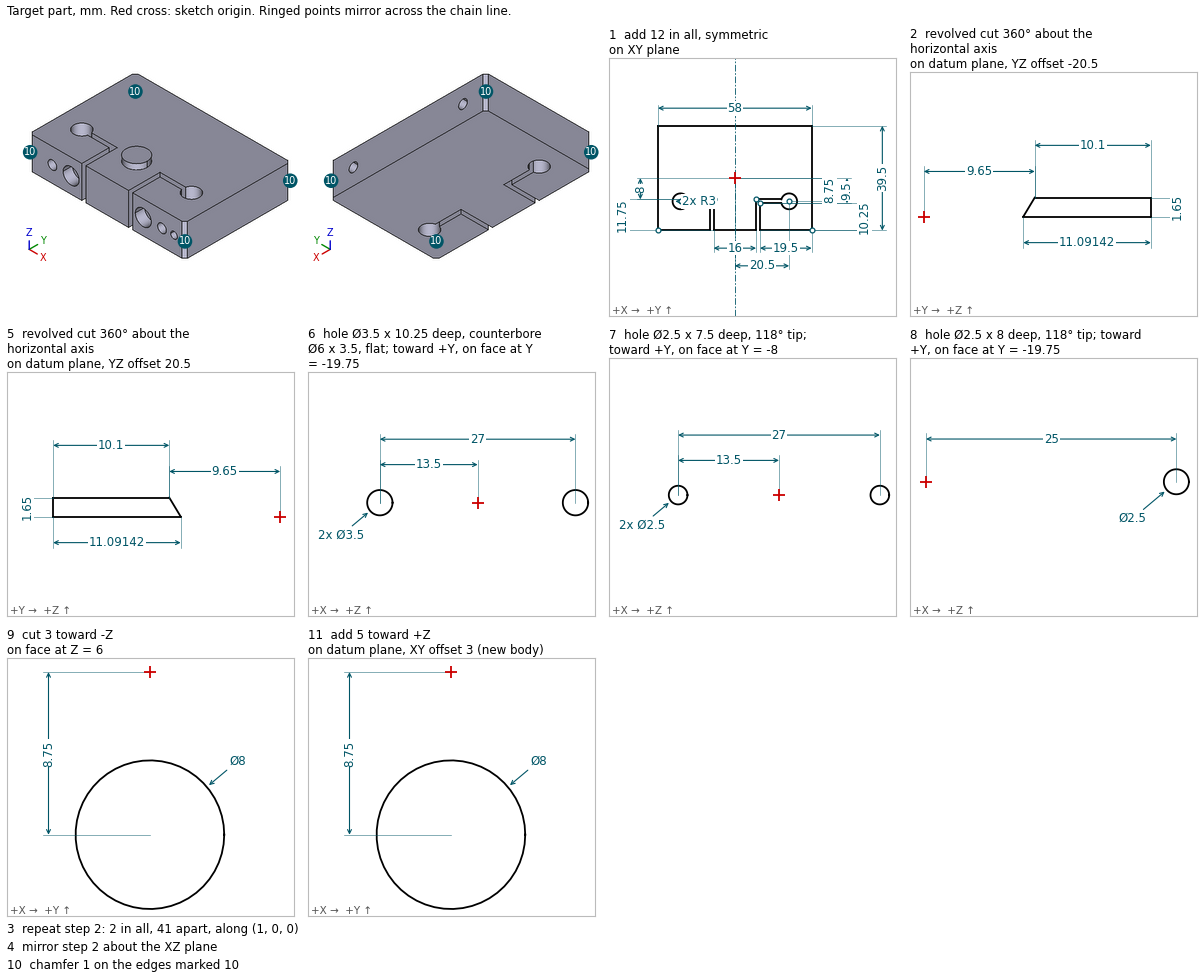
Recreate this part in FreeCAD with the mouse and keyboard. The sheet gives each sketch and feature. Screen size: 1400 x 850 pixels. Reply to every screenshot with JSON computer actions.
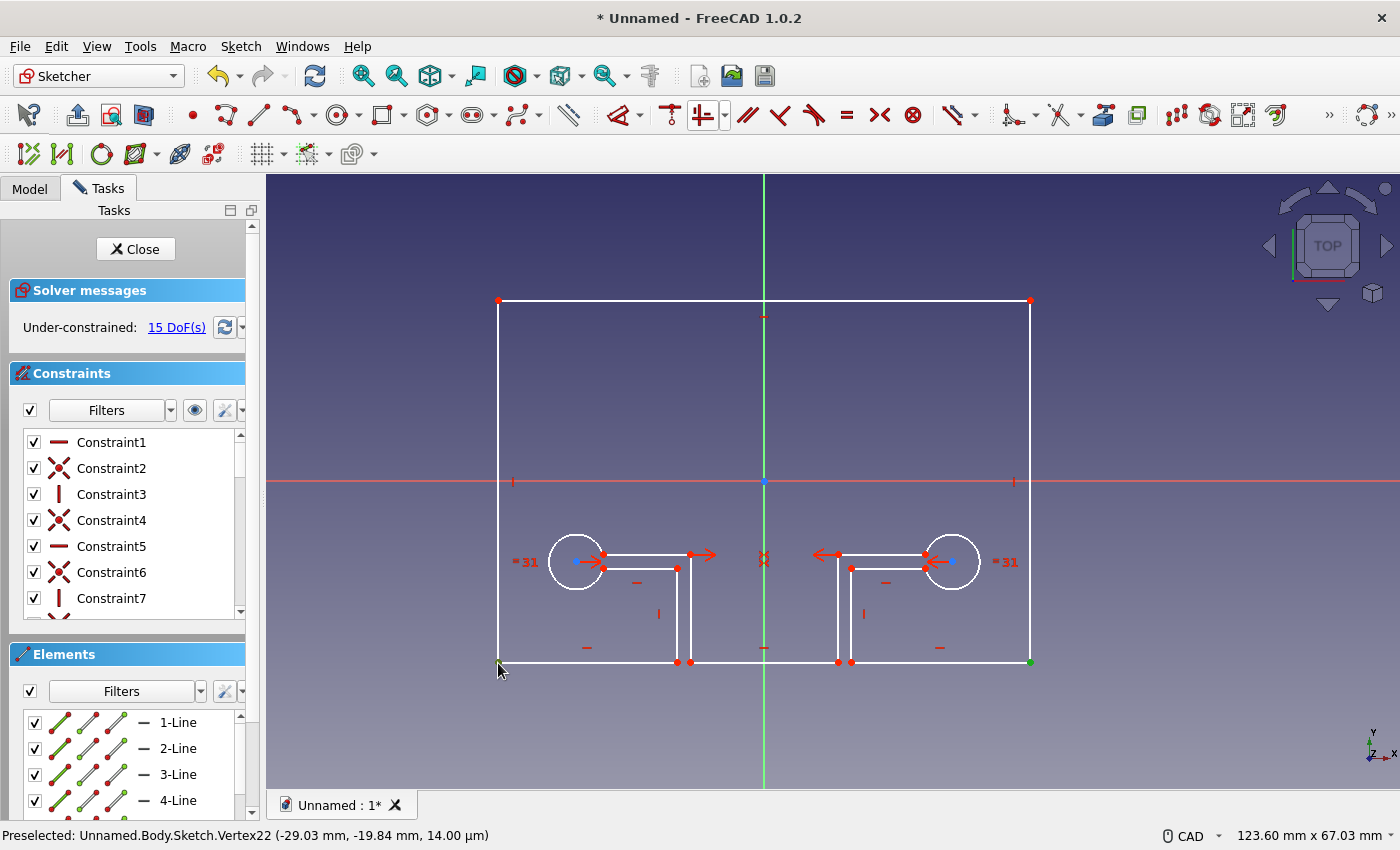
{"action": "left_click", "coordinate": [764, 721]}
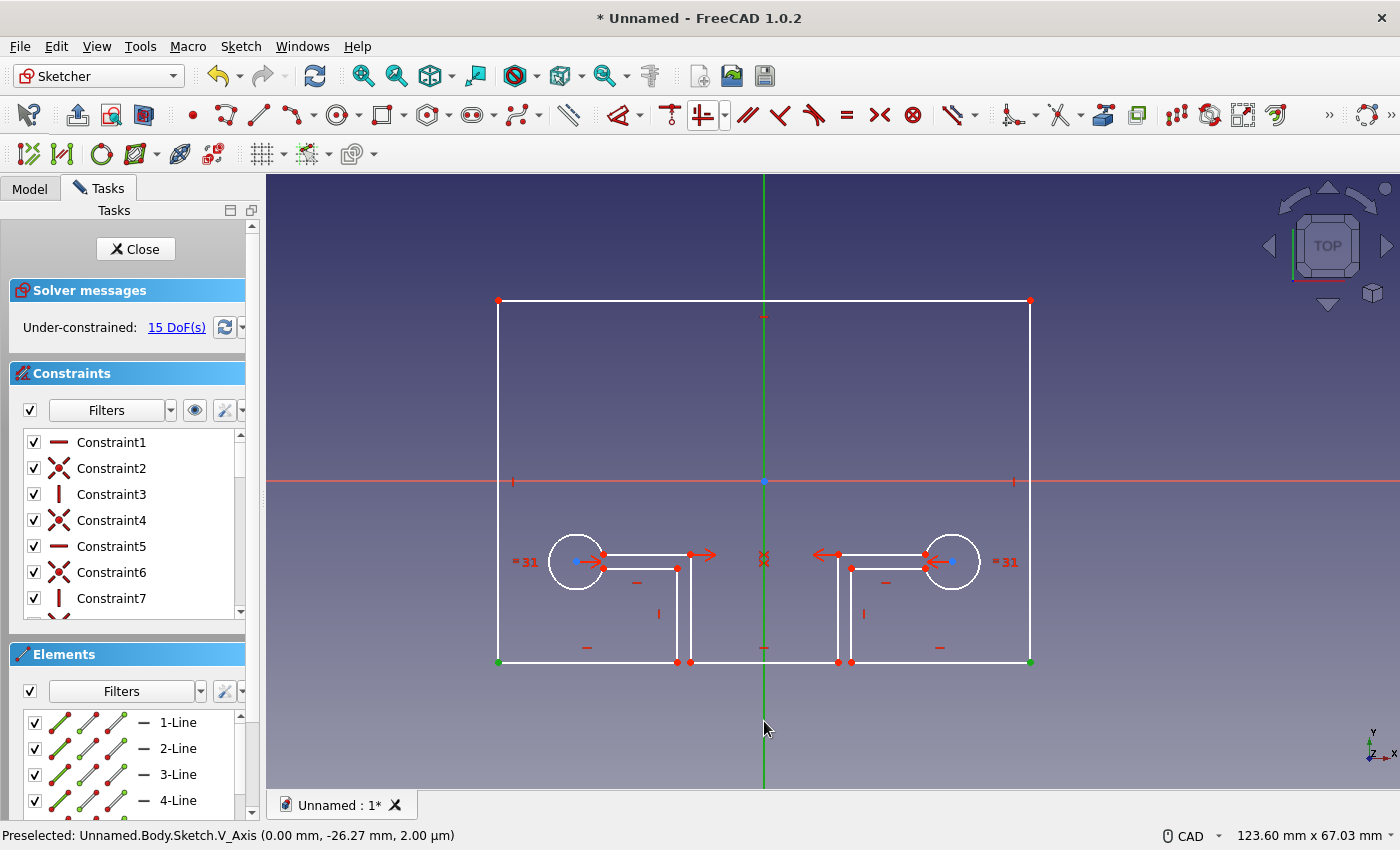
{"action": "left_click", "coordinate": [880, 116]}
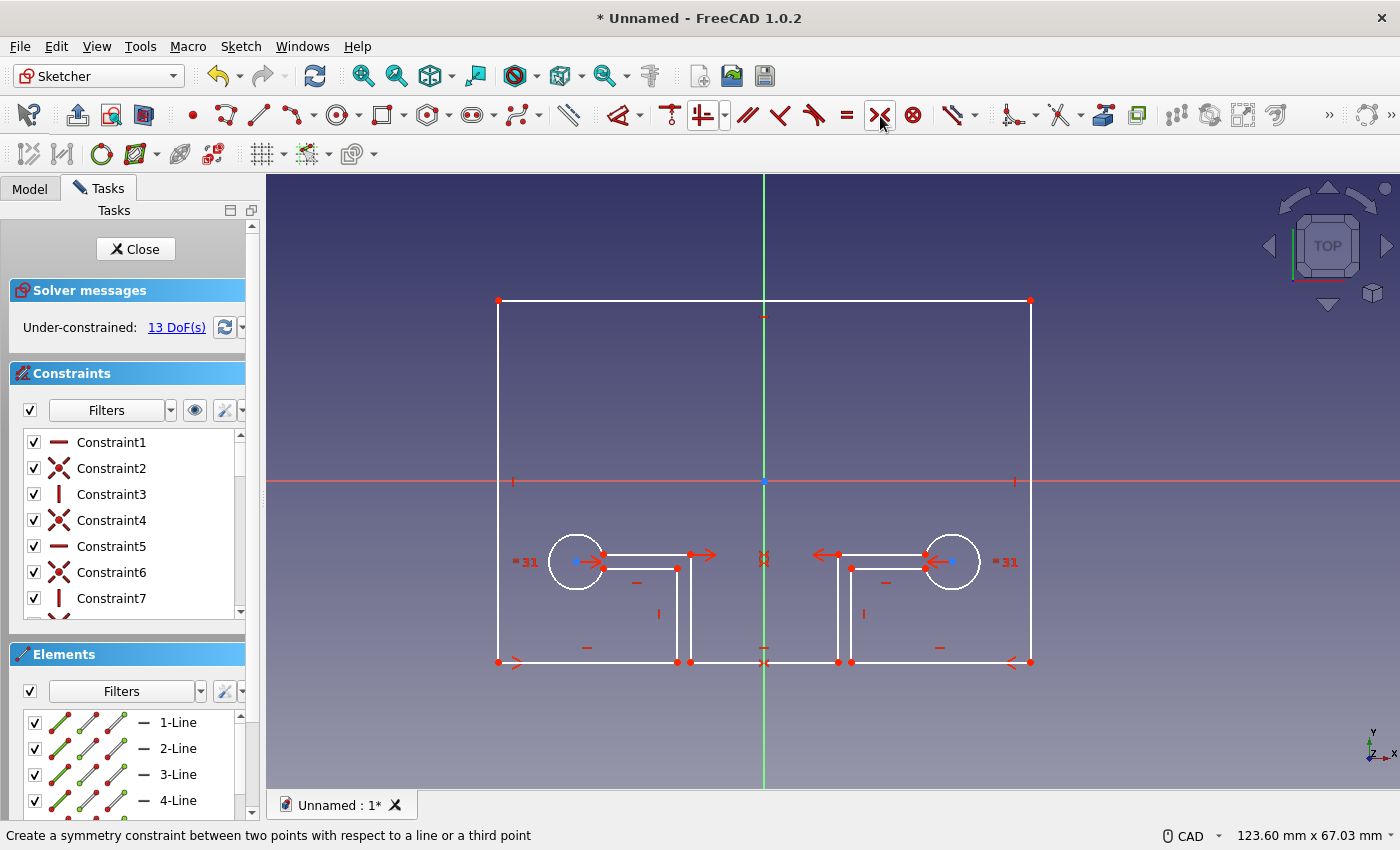
{"action": "left_click", "coordinate": [851, 569]}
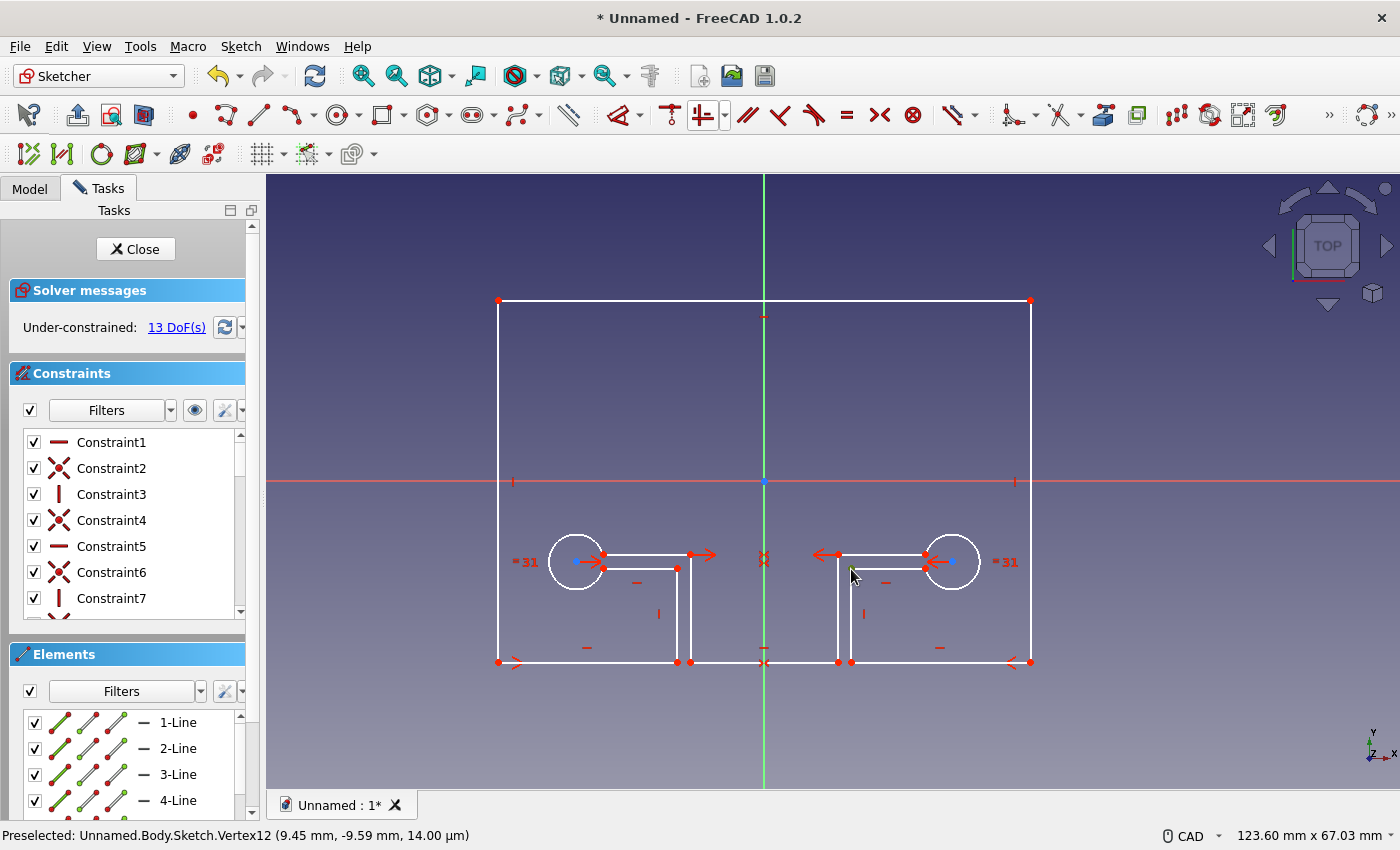
{"action": "left_click", "coordinate": [677, 569]}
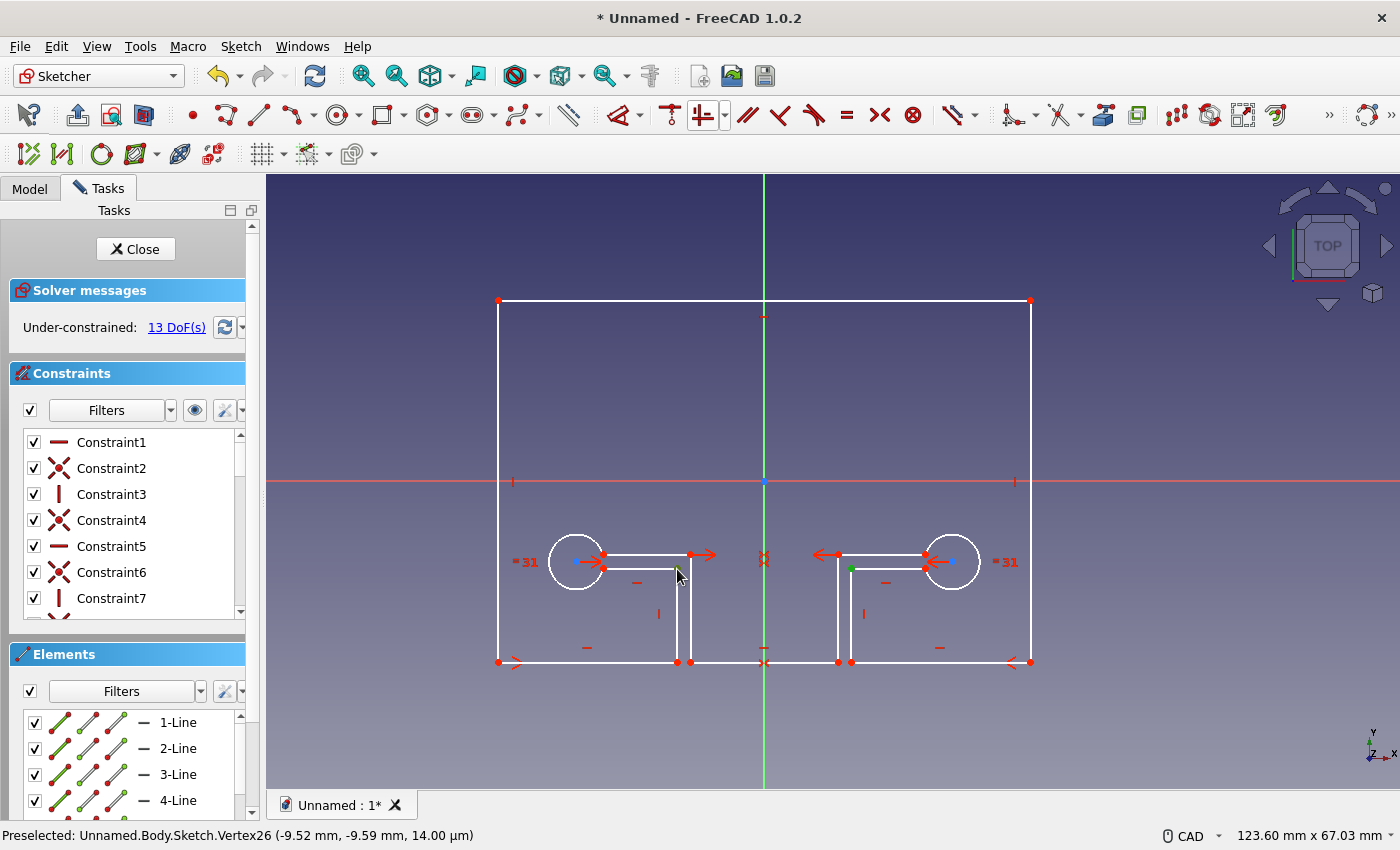
{"action": "left_click", "coordinate": [764, 721]}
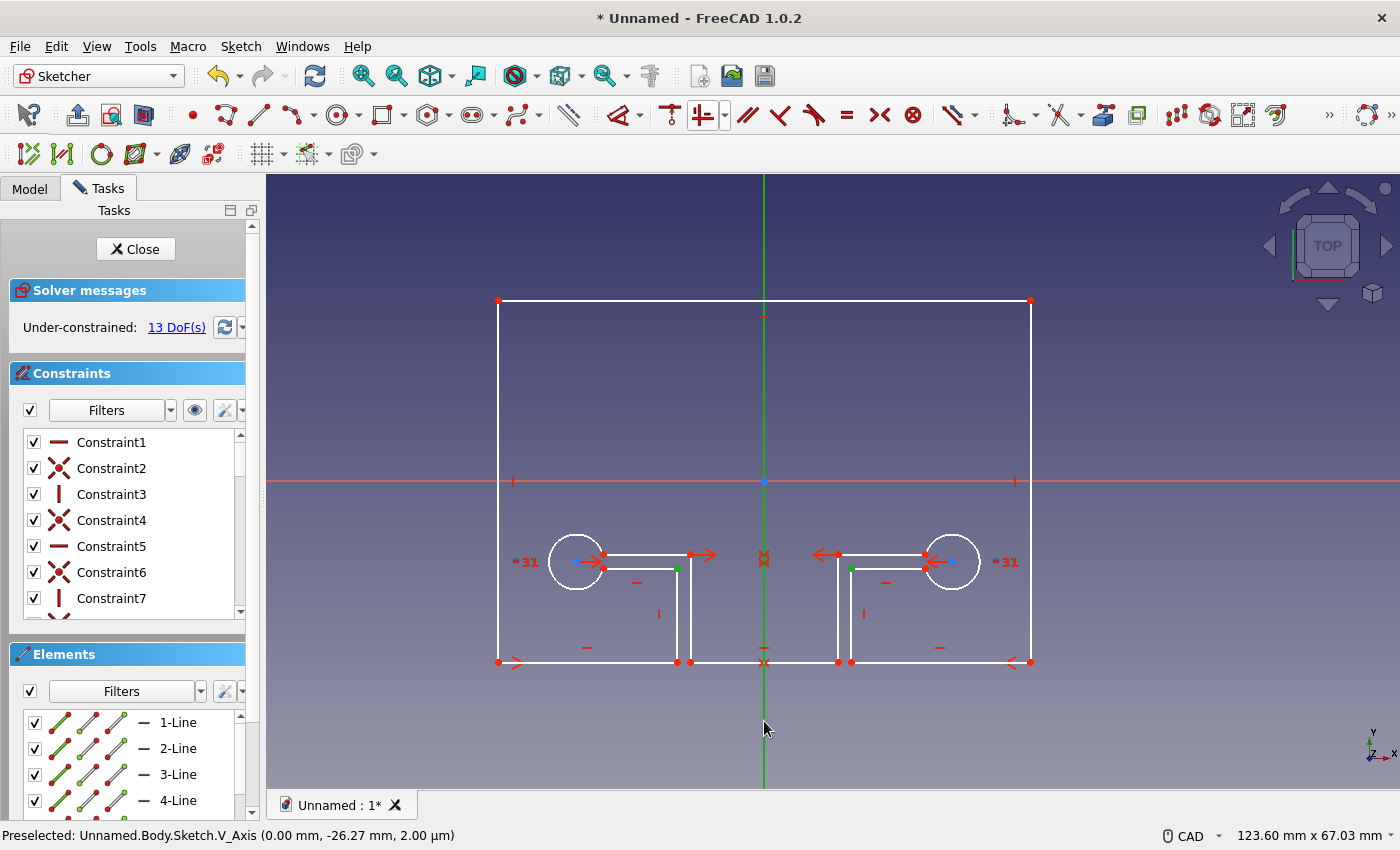
{"action": "key", "text": "s"}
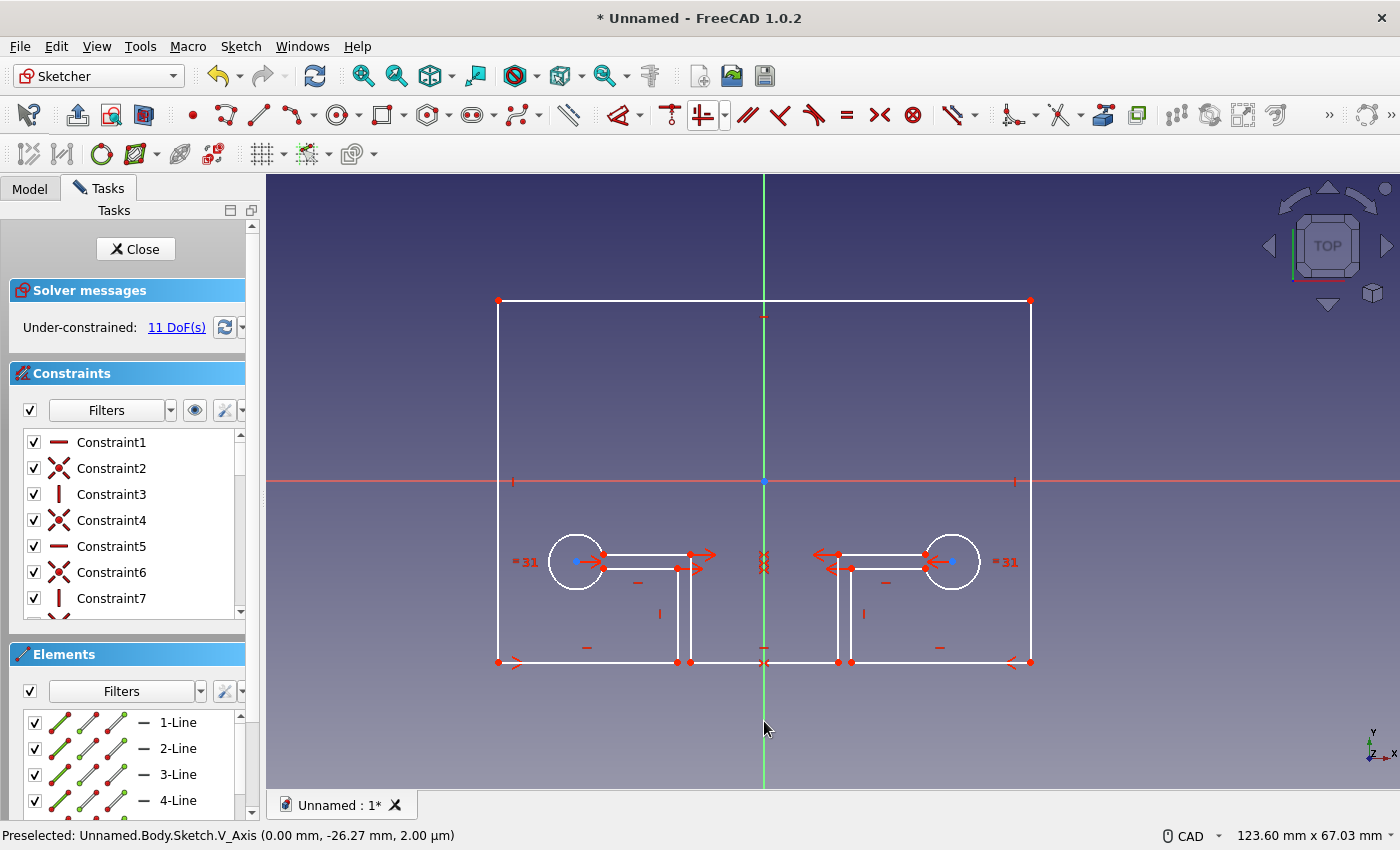
{"action": "left_click", "coordinate": [618, 116]}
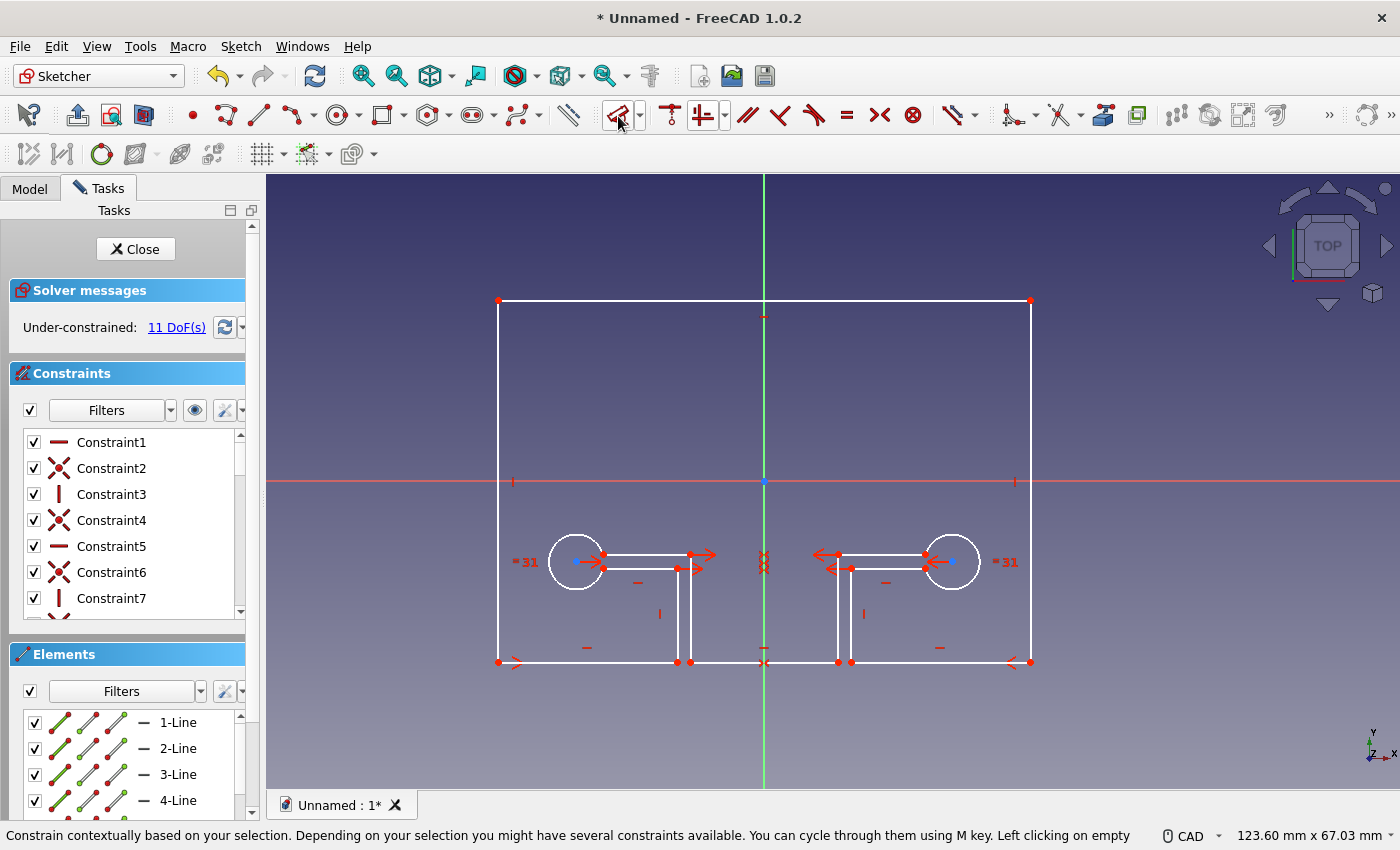
{"action": "scroll", "coordinate": [963, 587], "scroll_direction": "up", "scroll_amount": 2}